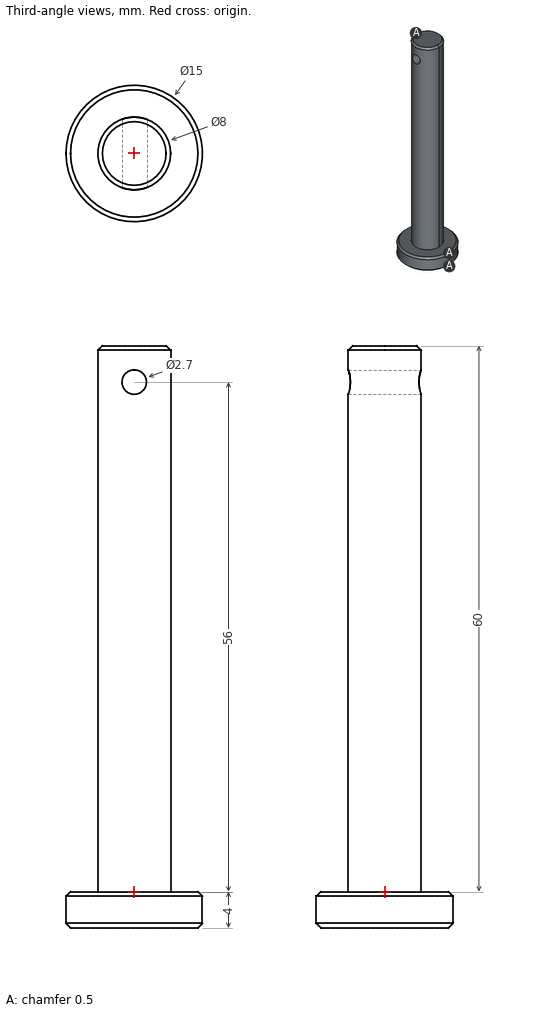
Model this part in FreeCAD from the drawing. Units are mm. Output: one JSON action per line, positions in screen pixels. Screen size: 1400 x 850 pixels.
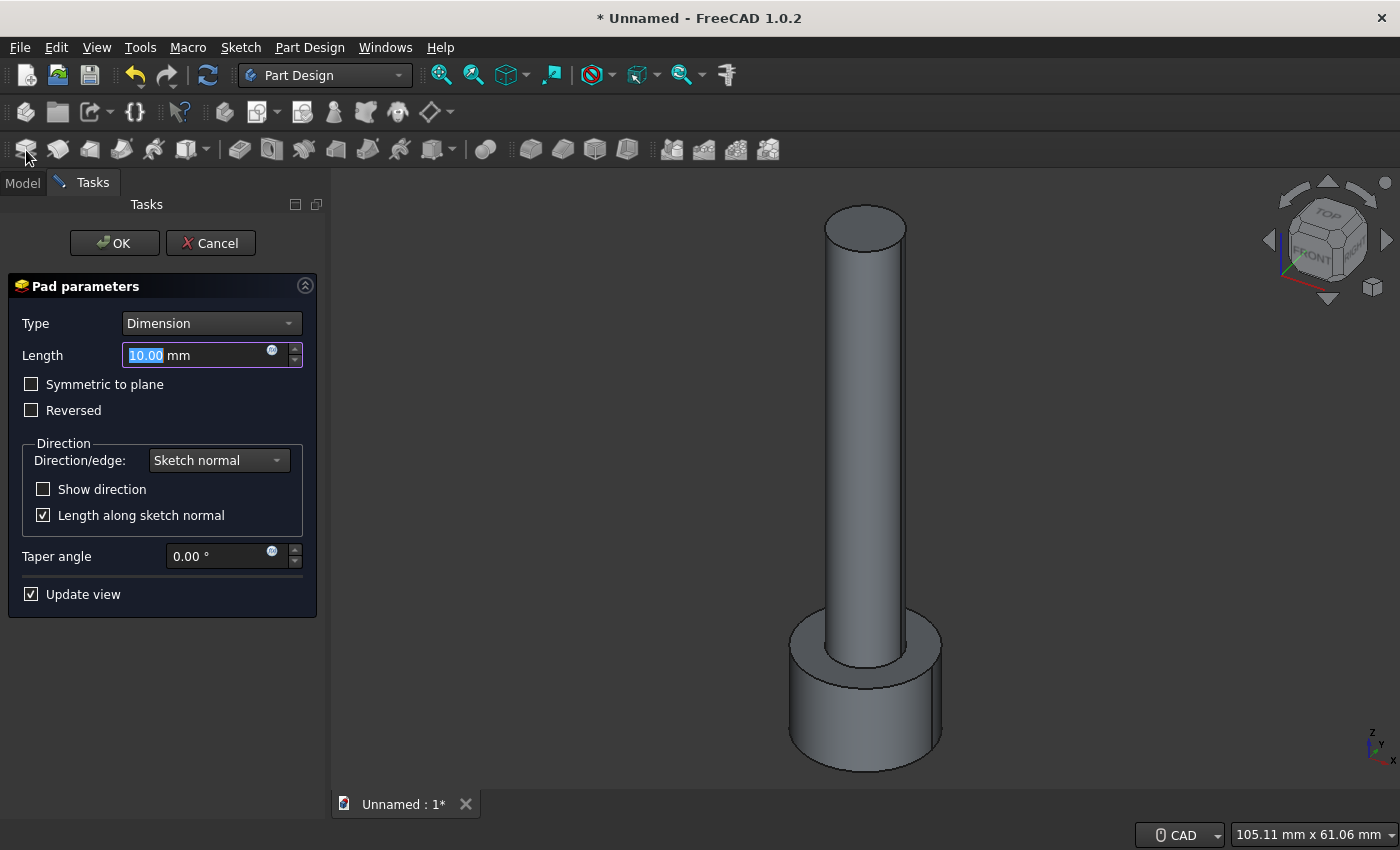
{"action": "type", "text": "4"}
{"action": "key", "text": "Tab"}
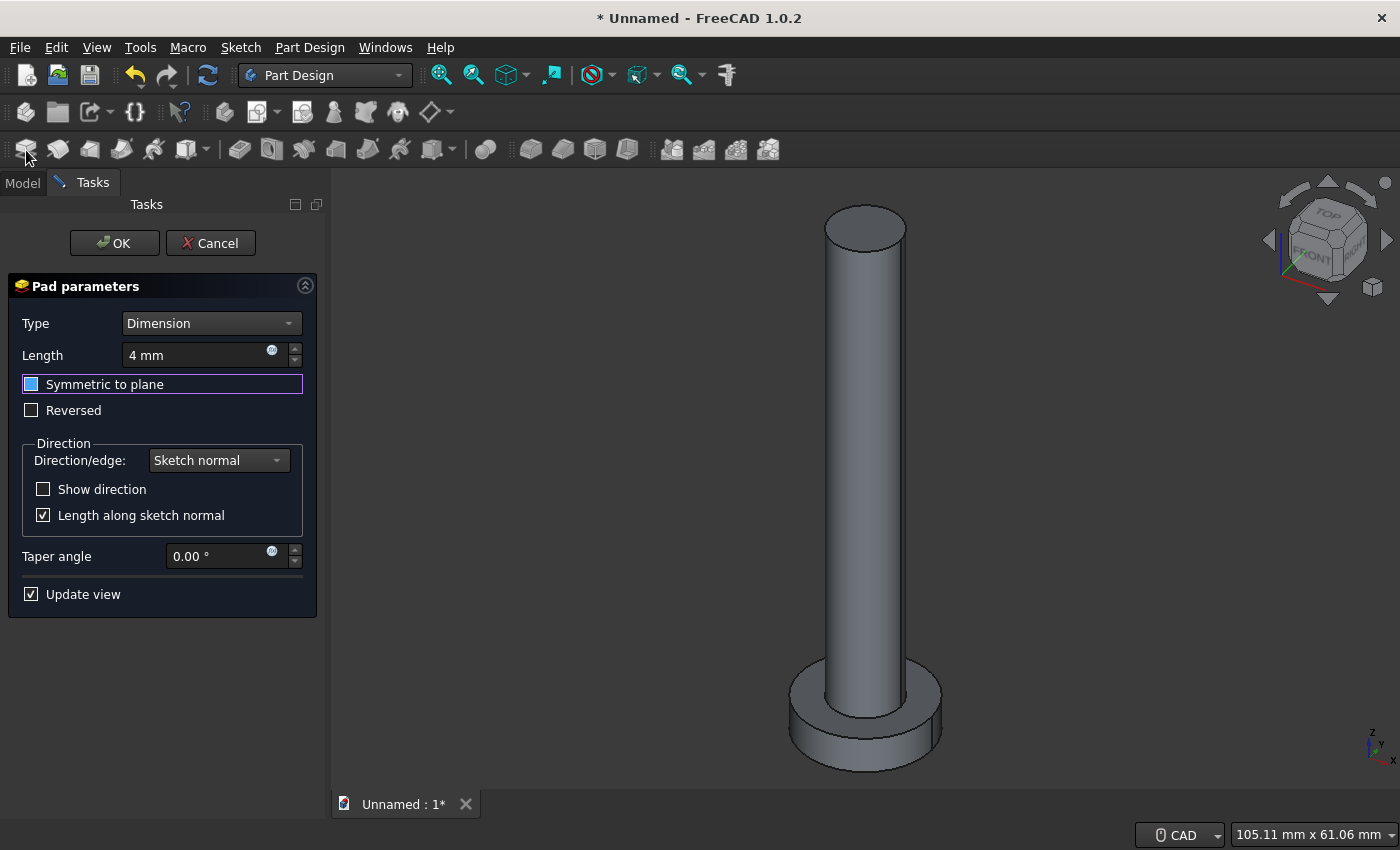
{"action": "left_click", "coordinate": [30, 410]}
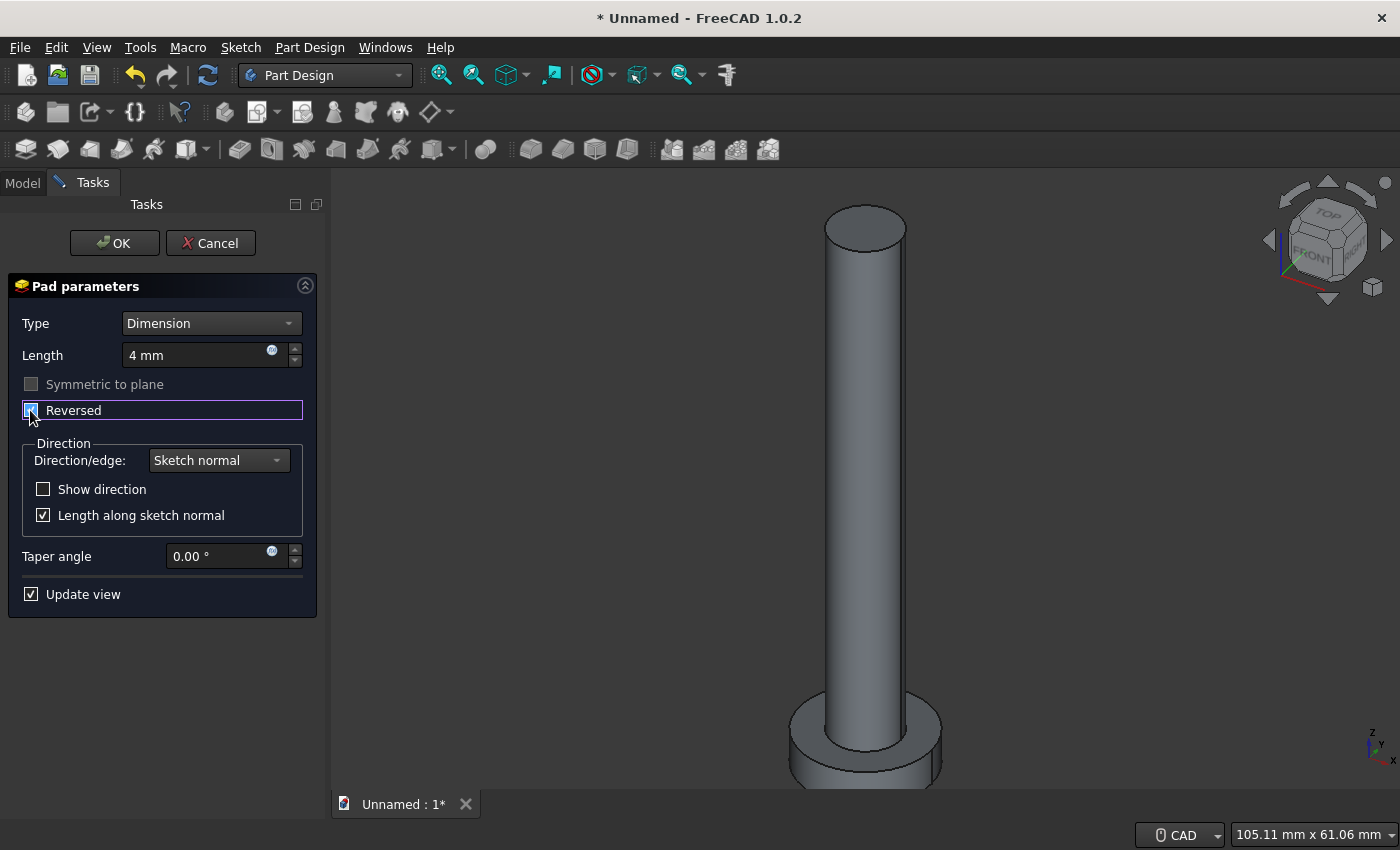
{"action": "left_click", "coordinate": [115, 243]}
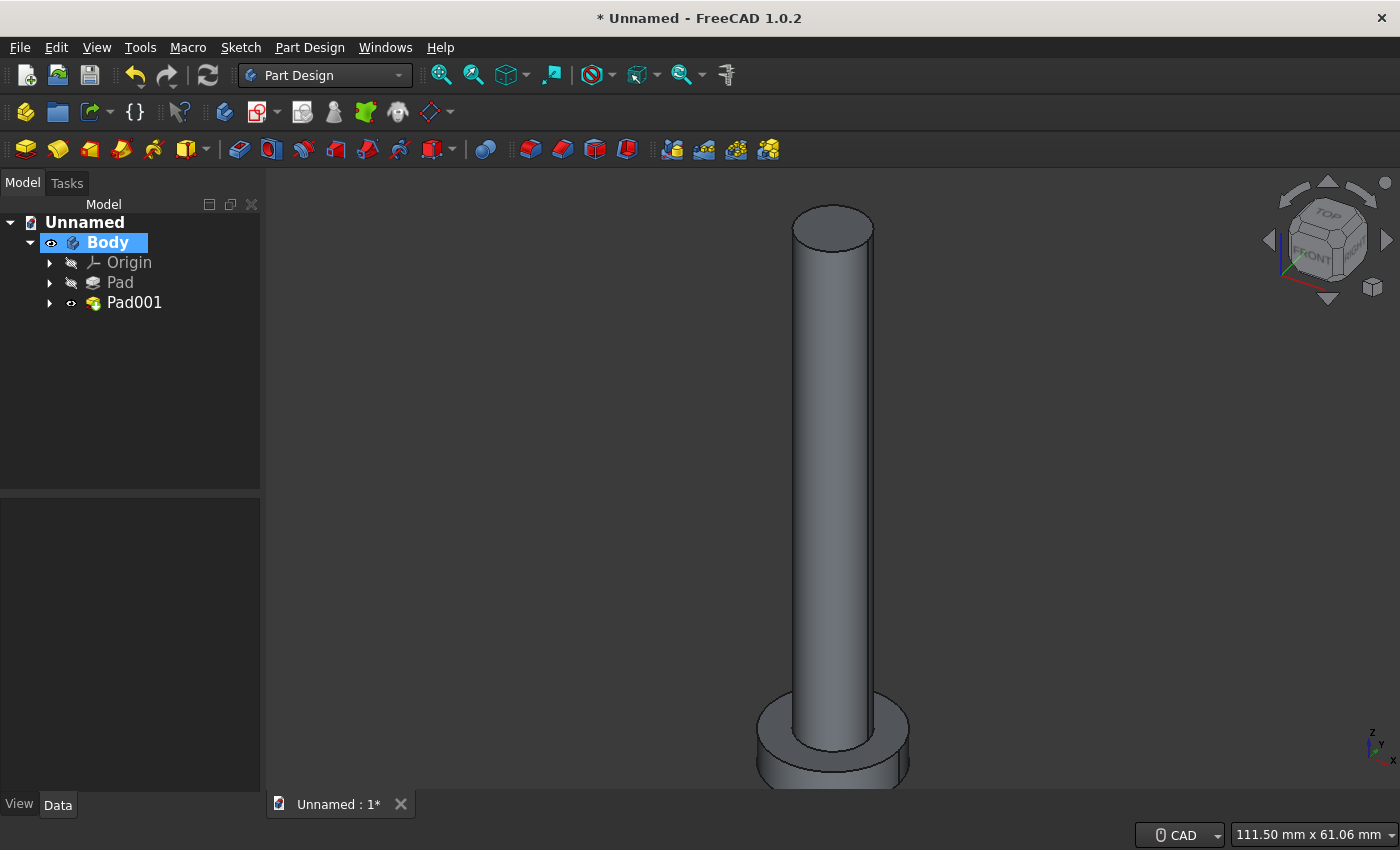
{"action": "left_click", "coordinate": [442, 76]}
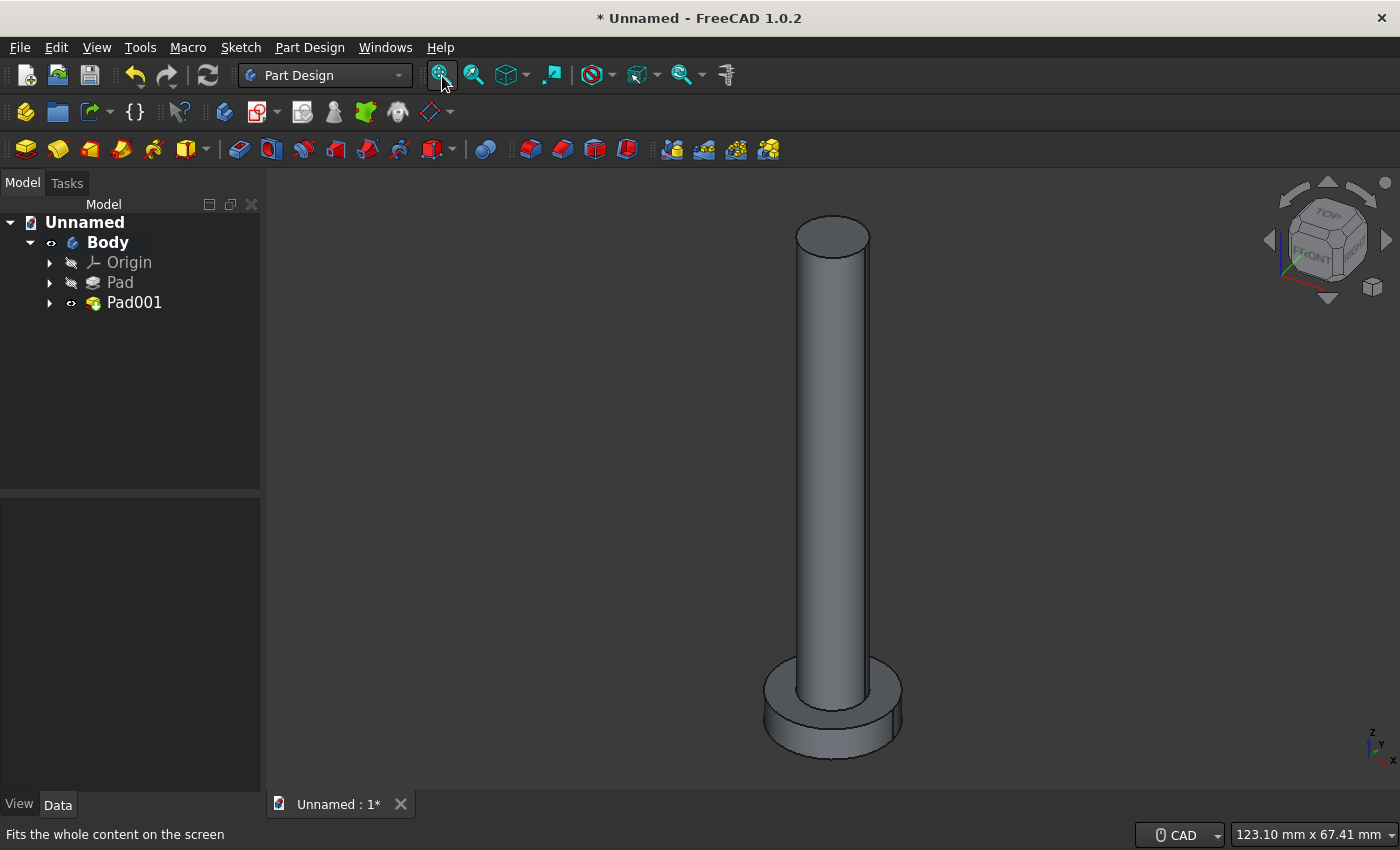
{"action": "left_click", "coordinate": [258, 112]}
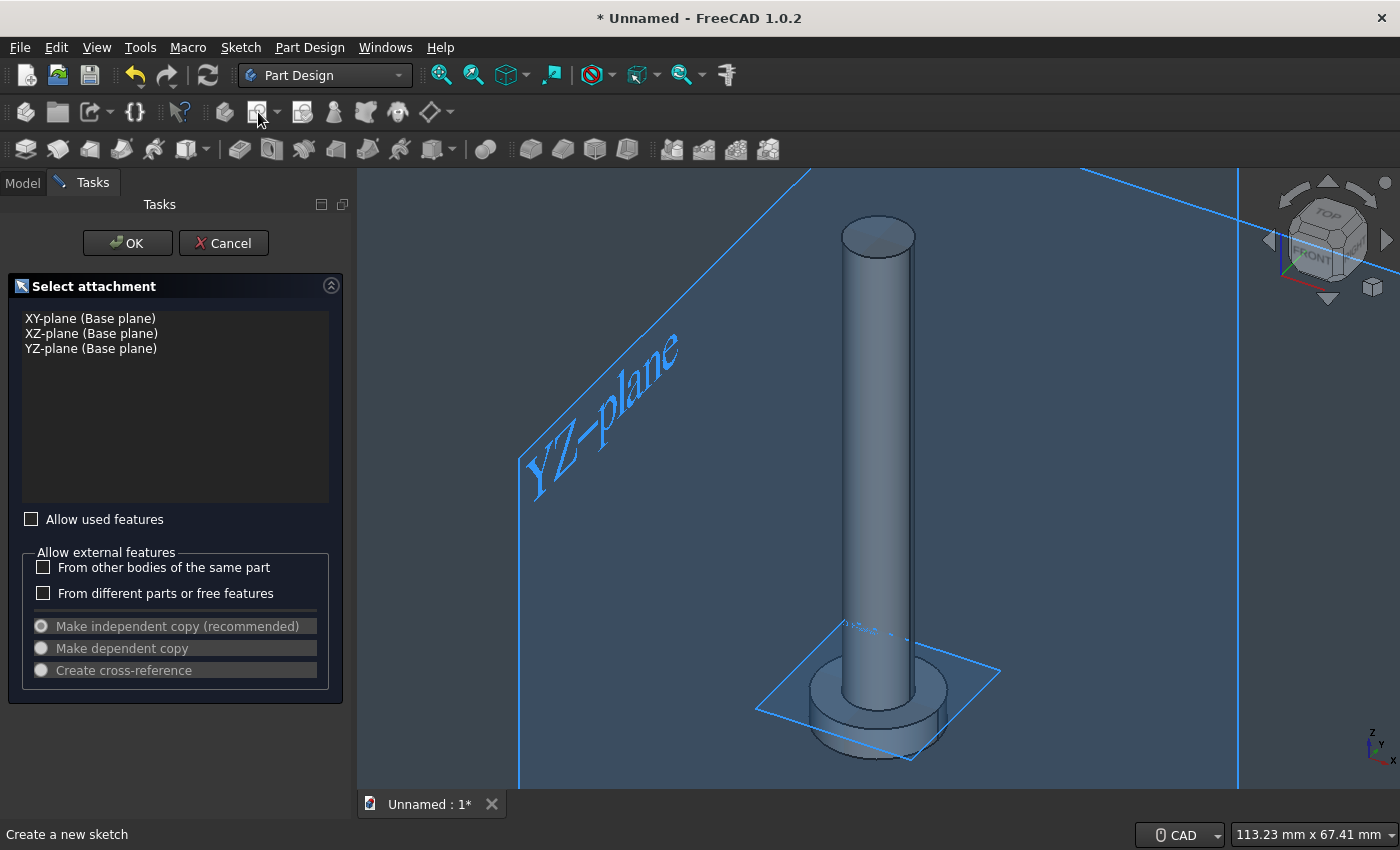
{"action": "left_click", "coordinate": [82, 334]}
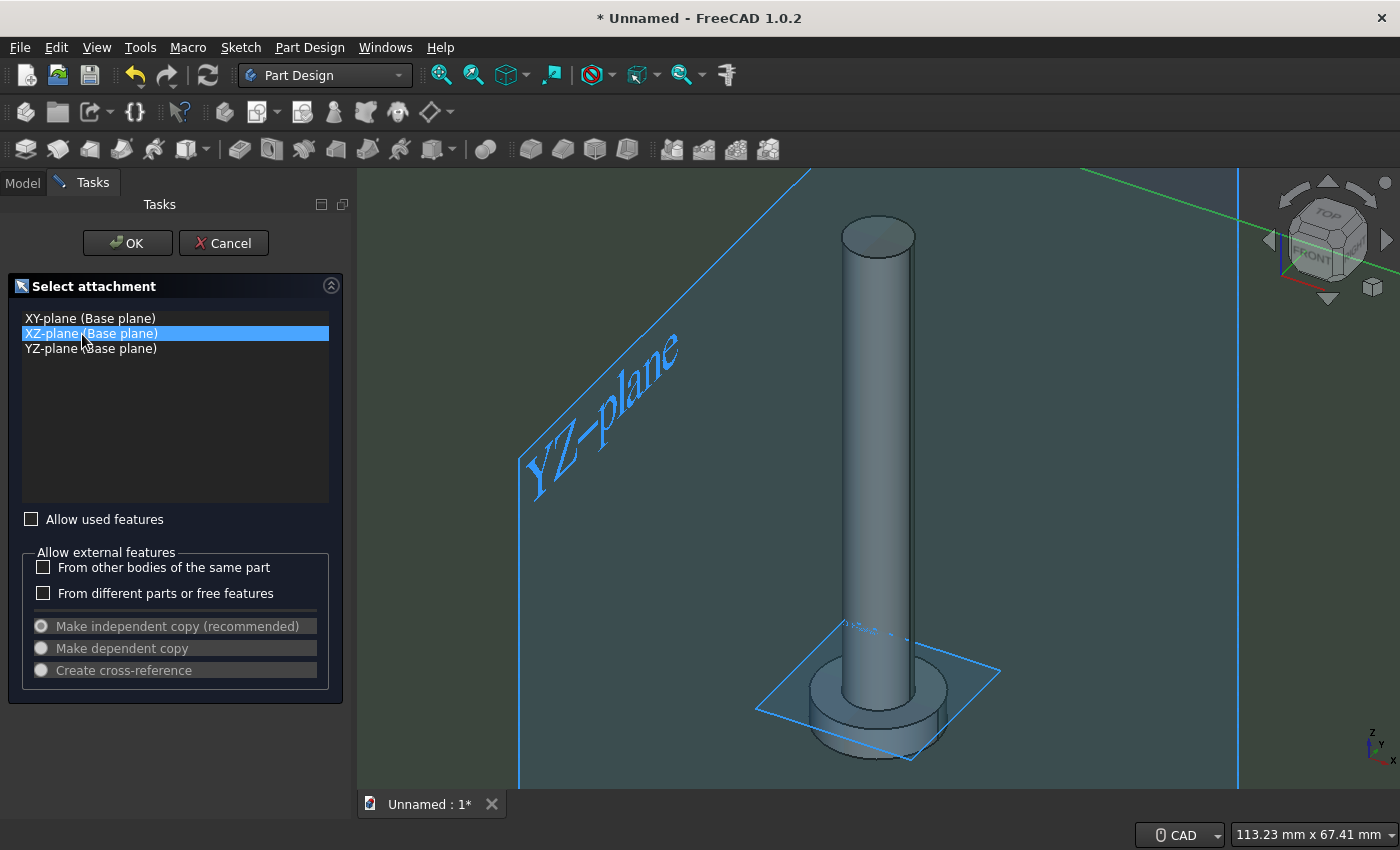
{"action": "left_click", "coordinate": [128, 243]}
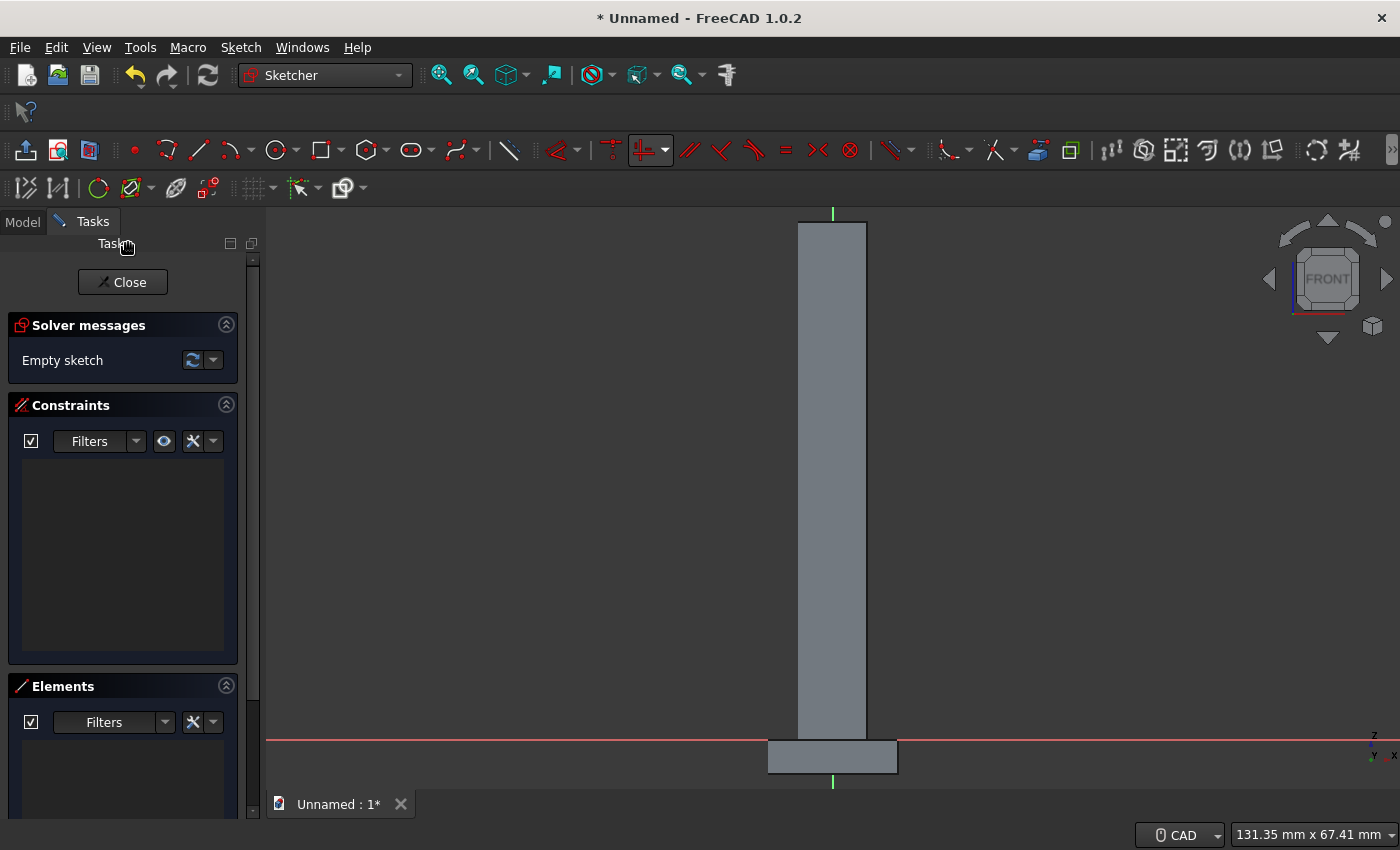
{"action": "left_click", "coordinate": [90, 150]}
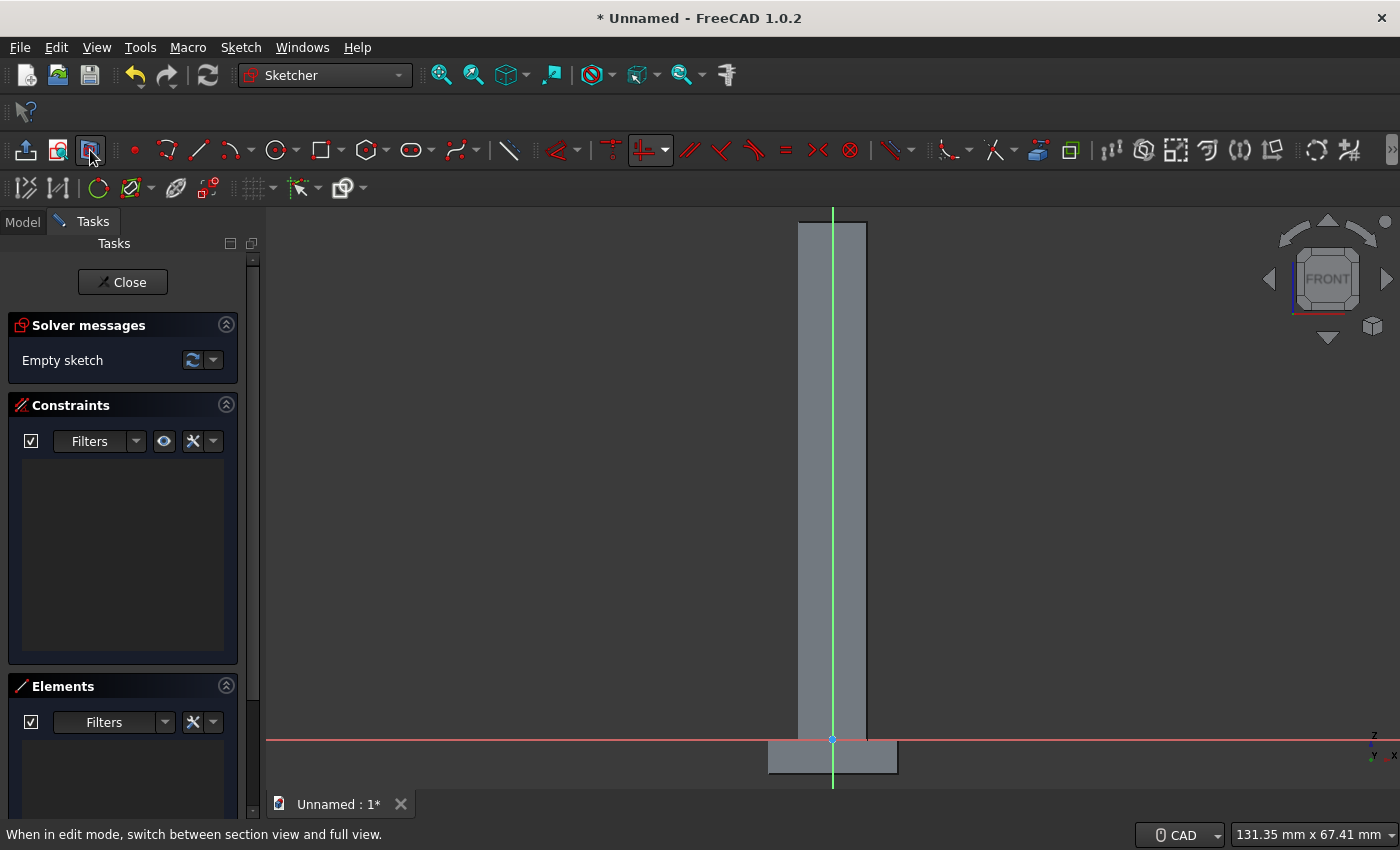
{"action": "scroll", "coordinate": [837, 241], "scroll_direction": "up", "scroll_amount": 14}